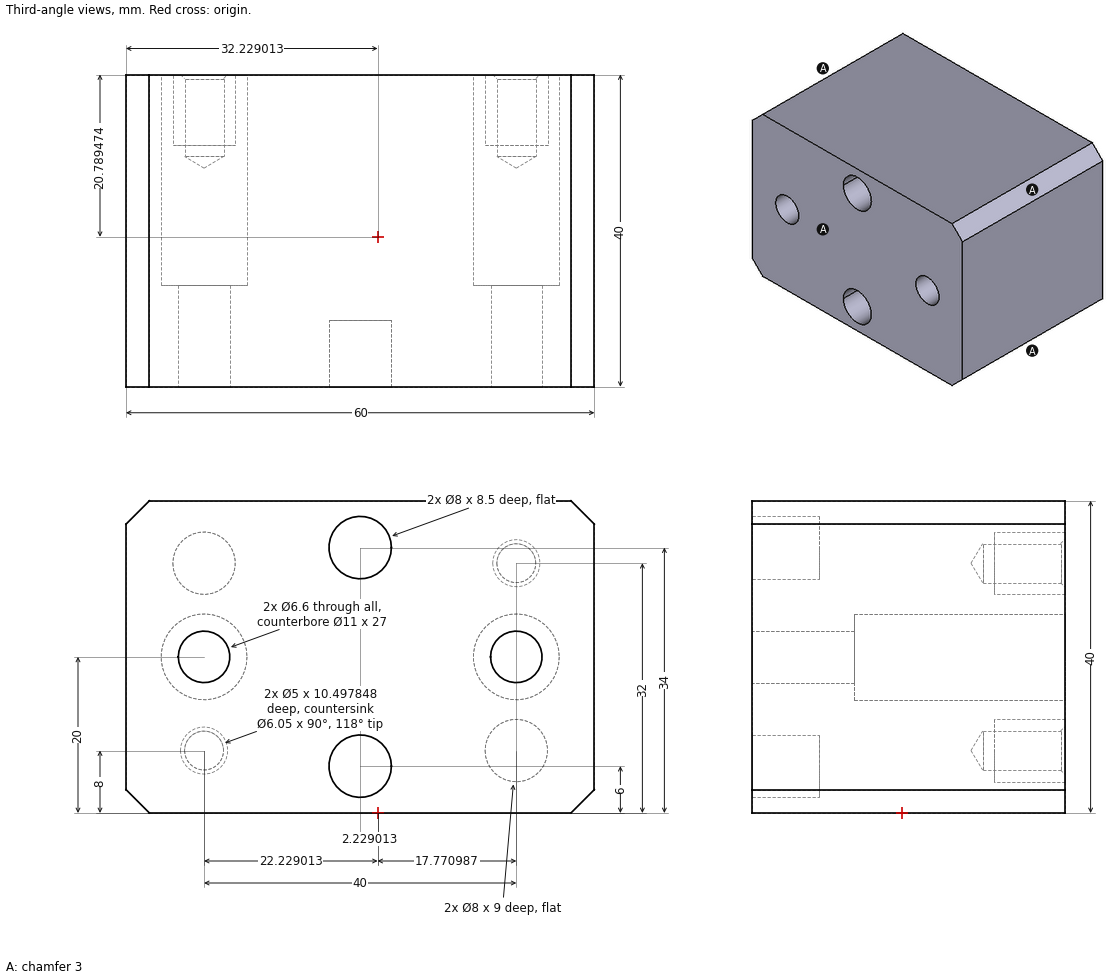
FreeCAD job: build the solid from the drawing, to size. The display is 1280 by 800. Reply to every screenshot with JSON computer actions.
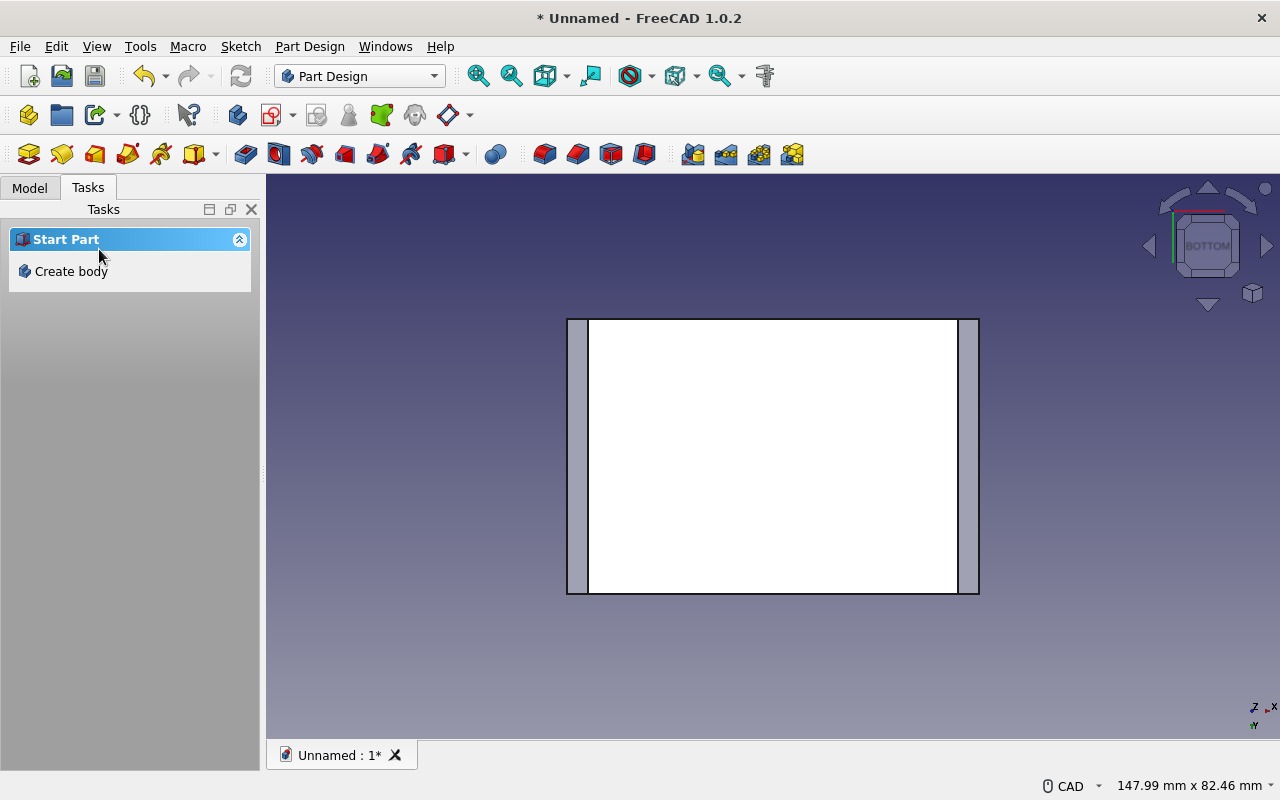
{"action": "key", "text": "4"}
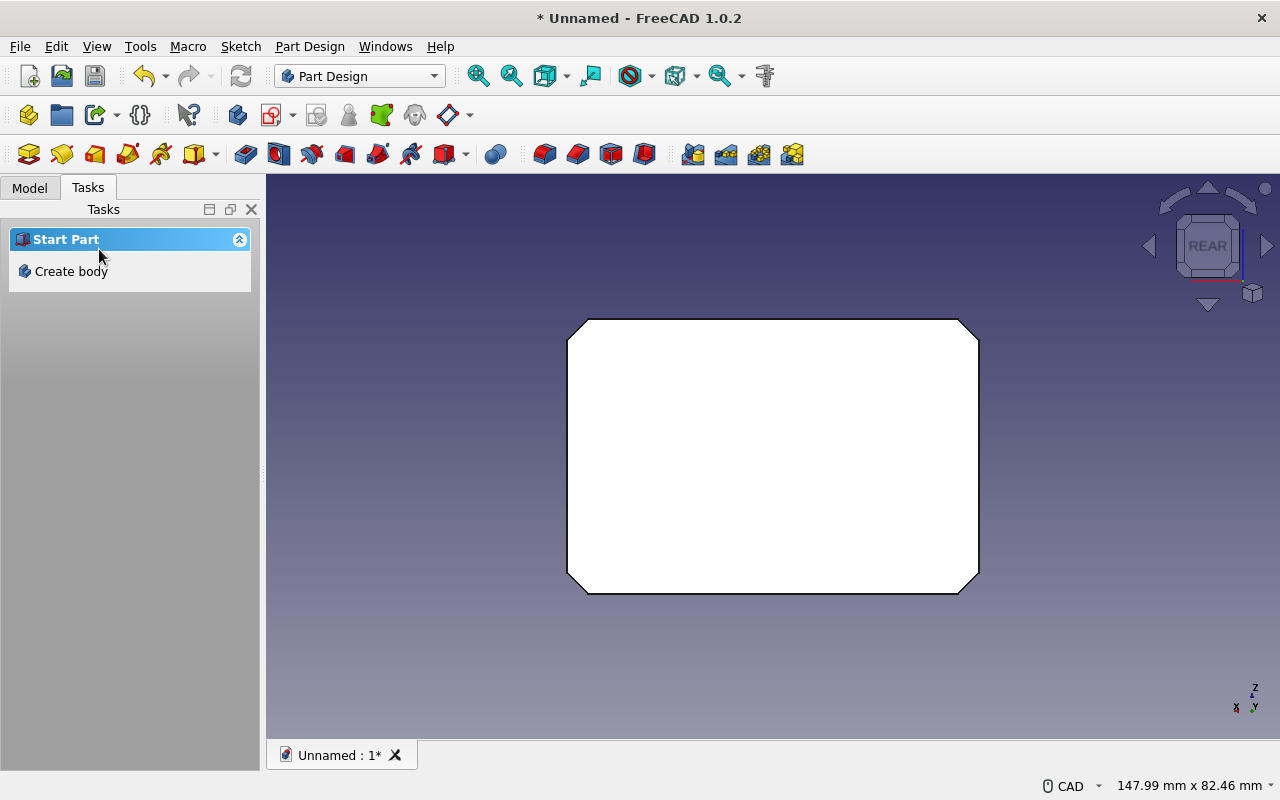
{"action": "left_click", "coordinate": [714, 455]}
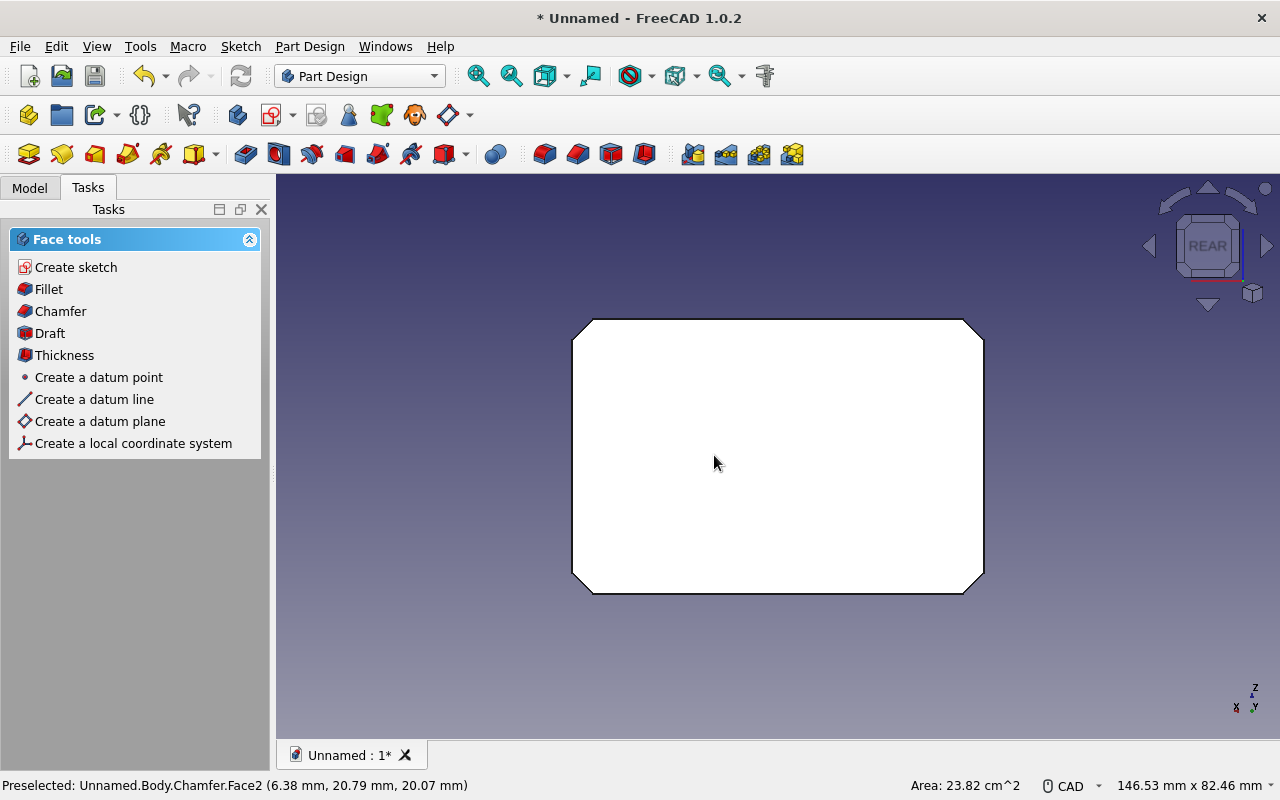
{"action": "left_click", "coordinate": [270, 116]}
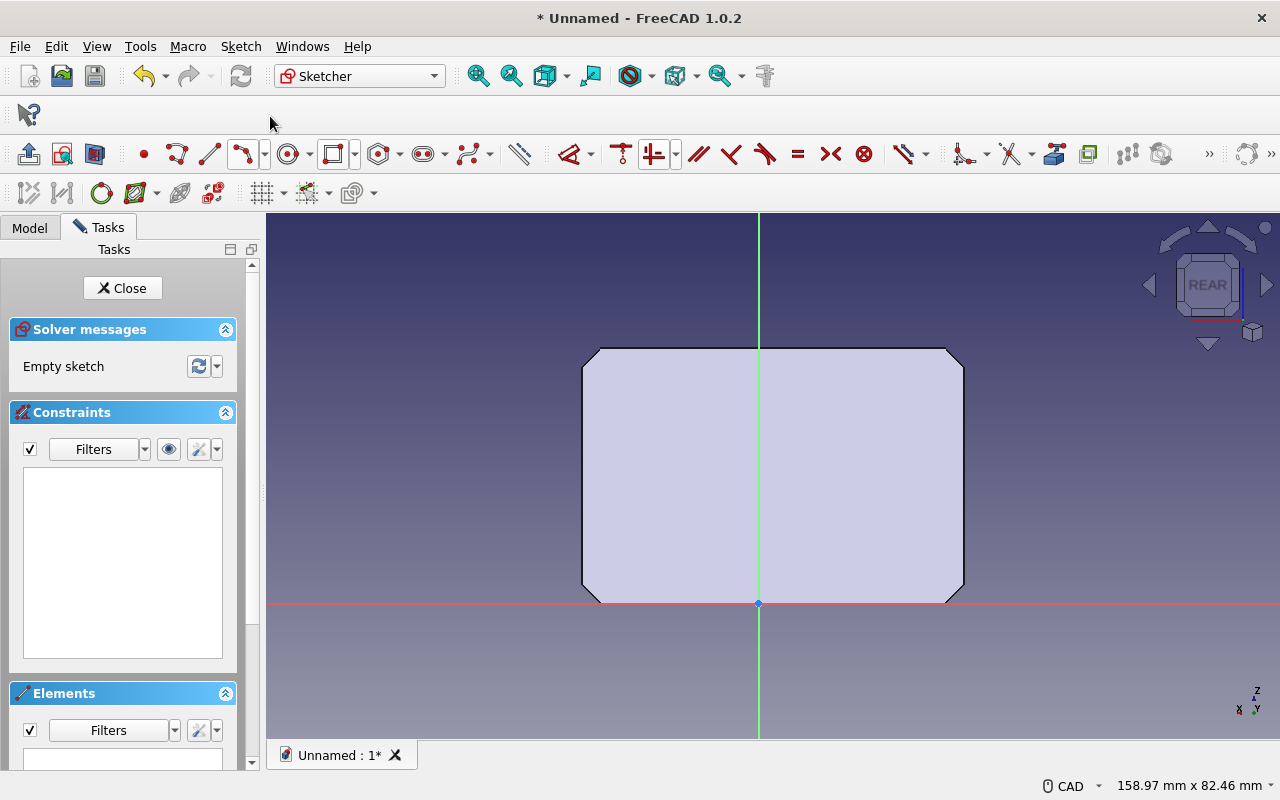
{"action": "scroll", "coordinate": [912, 529], "scroll_direction": "up", "scroll_amount": 2}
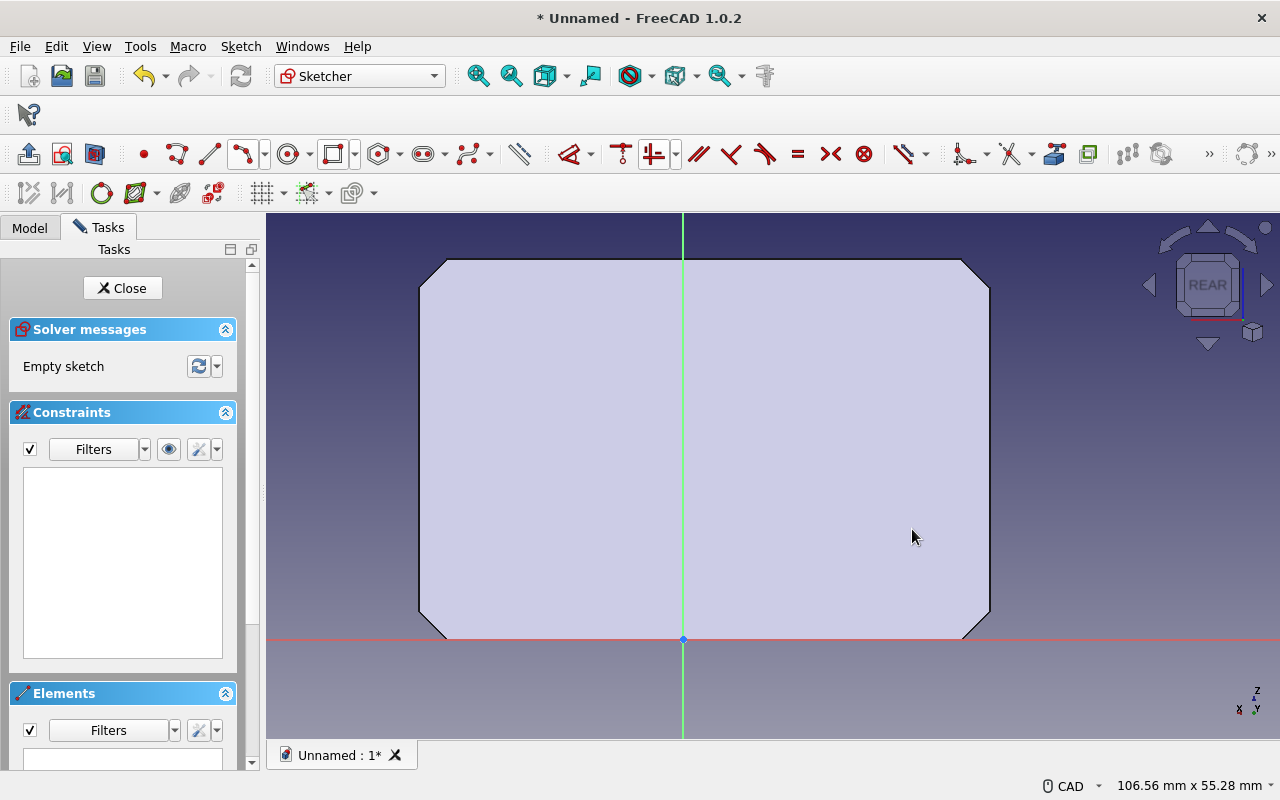
{"action": "left_click", "coordinate": [288, 154]}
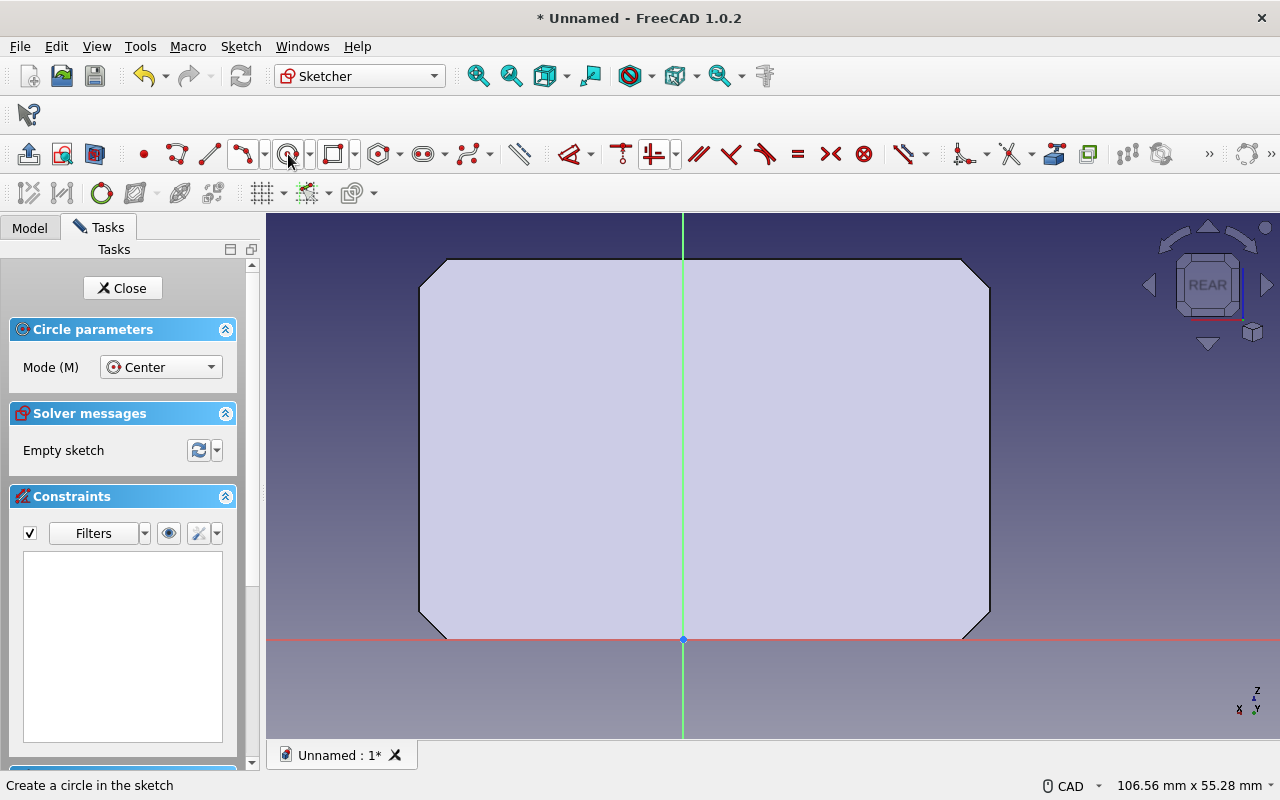
{"action": "left_click", "coordinate": [895, 564]}
{"action": "mouse_move", "coordinate": [911, 547]}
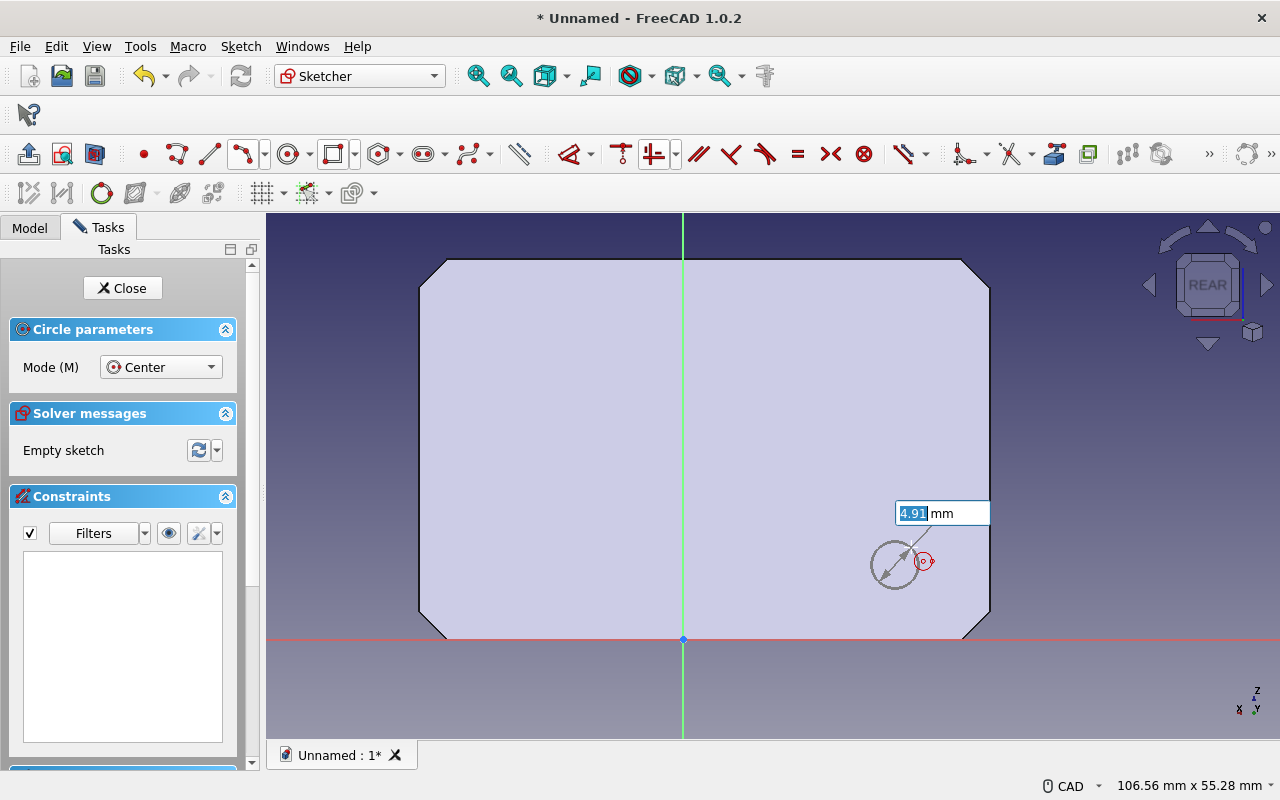
{"action": "type", "text": "5"}
{"action": "key", "text": "Return"}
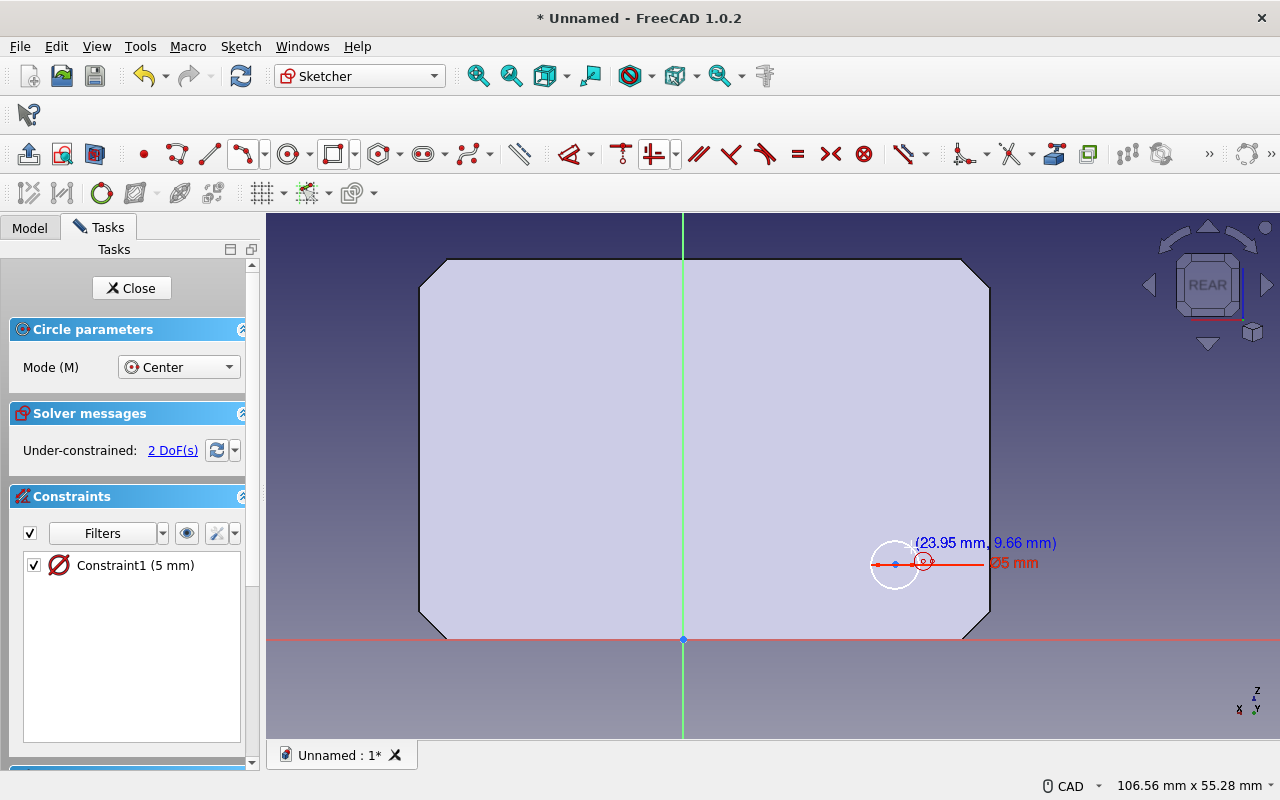
{"action": "left_click", "coordinate": [514, 335]}
{"action": "mouse_move", "coordinate": [531, 319]}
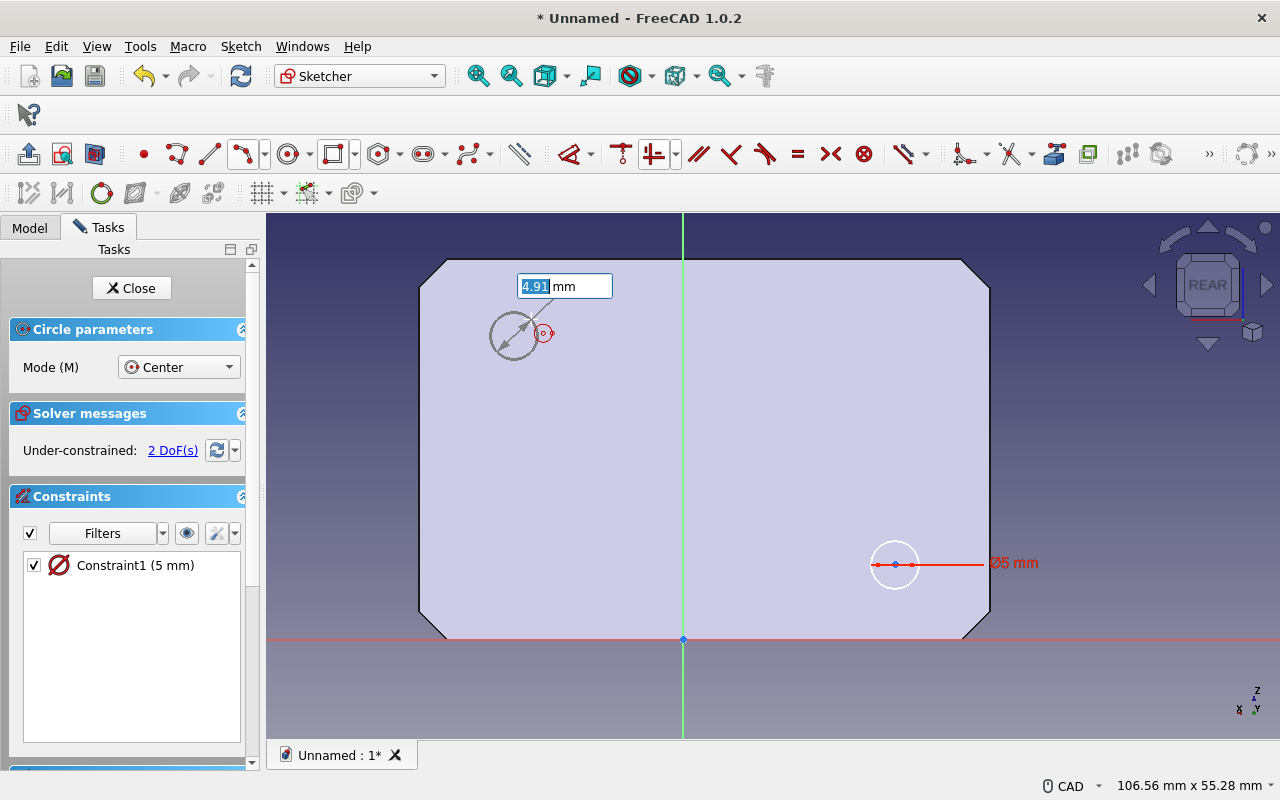
{"action": "type", "text": "5"}
{"action": "key", "text": "Return"}
{"action": "key", "text": "Escape"}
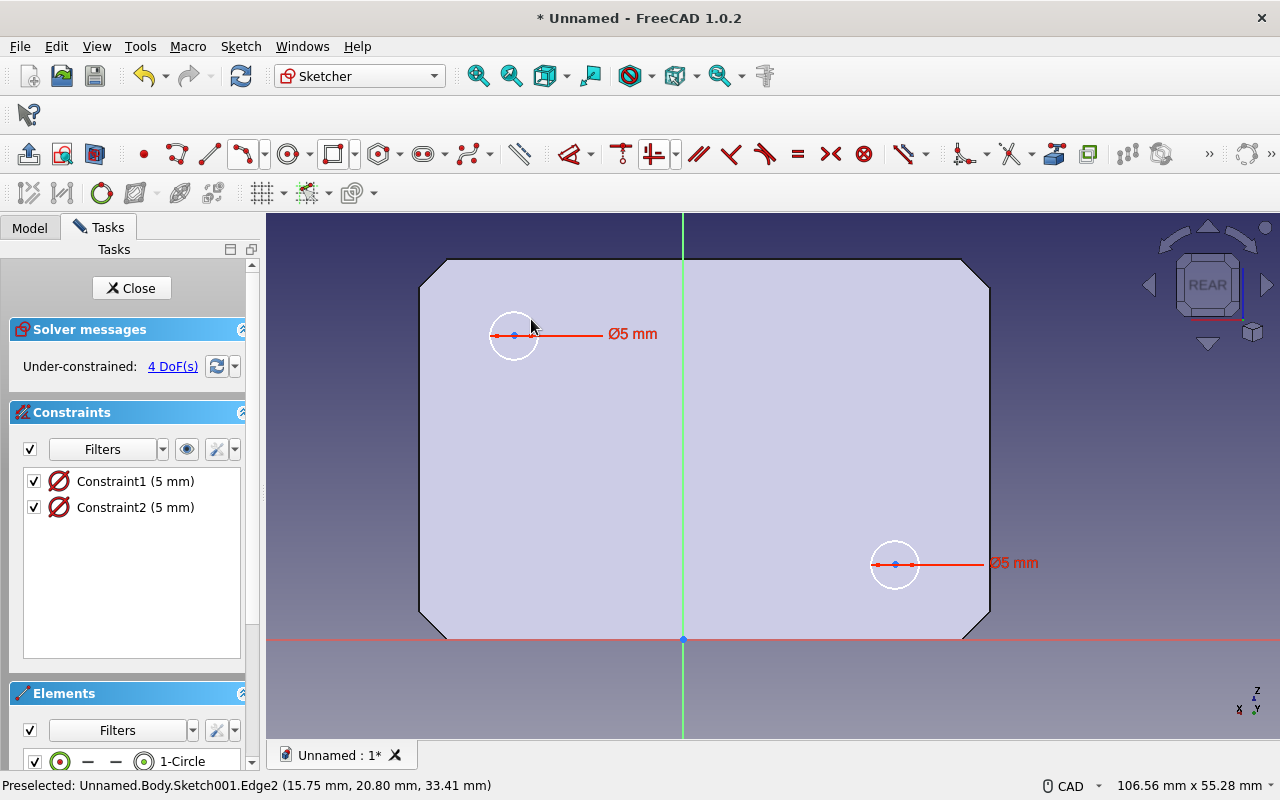
{"action": "key", "text": "d"}